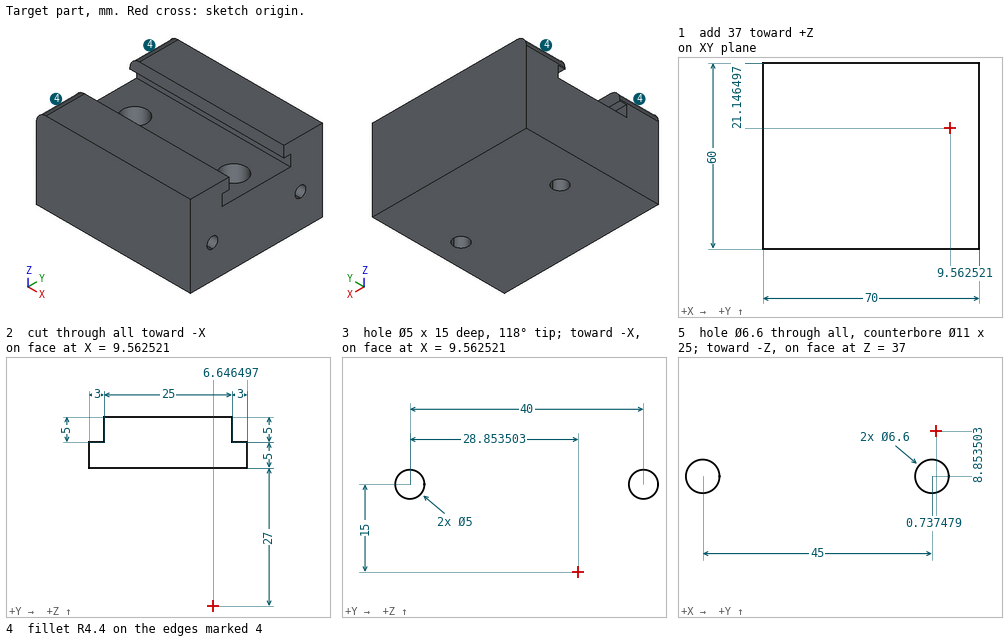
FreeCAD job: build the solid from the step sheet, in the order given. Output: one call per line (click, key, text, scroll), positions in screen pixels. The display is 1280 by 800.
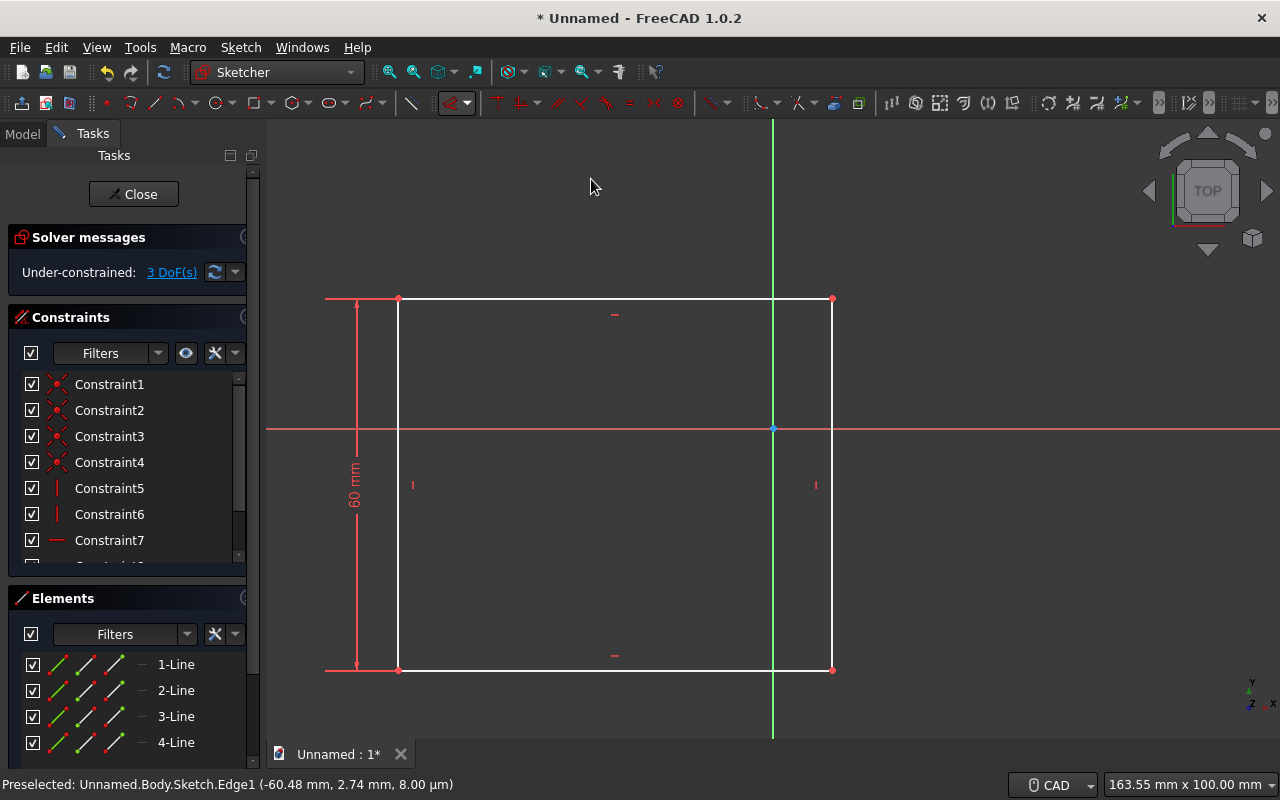
click(528, 671)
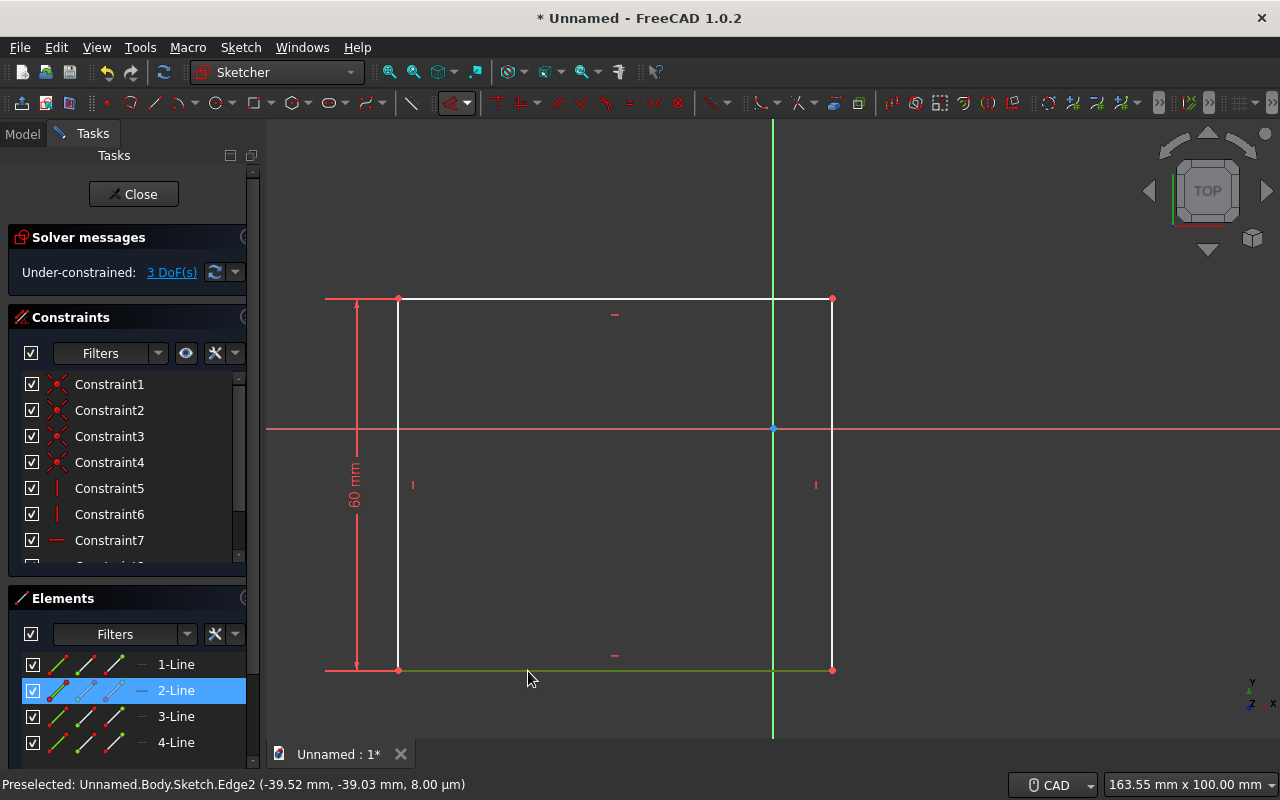
click(470, 104)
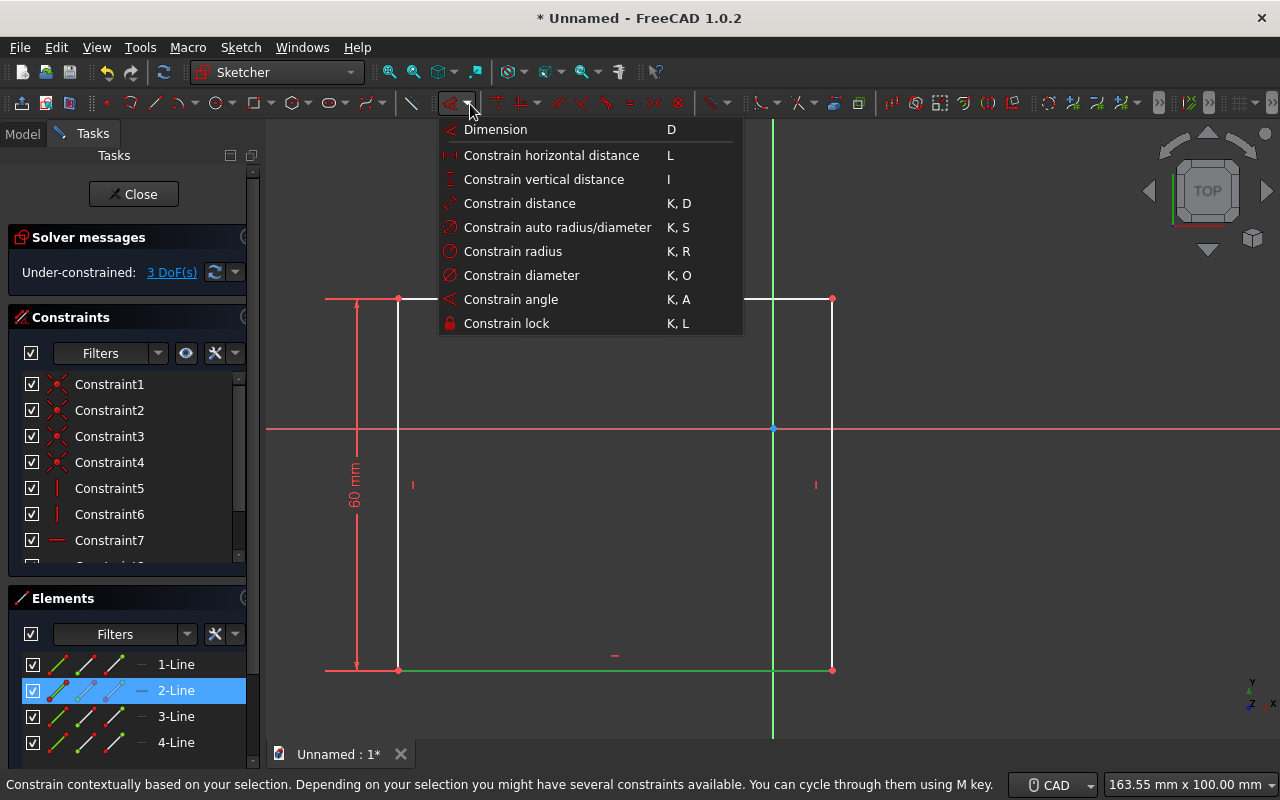
click(591, 155)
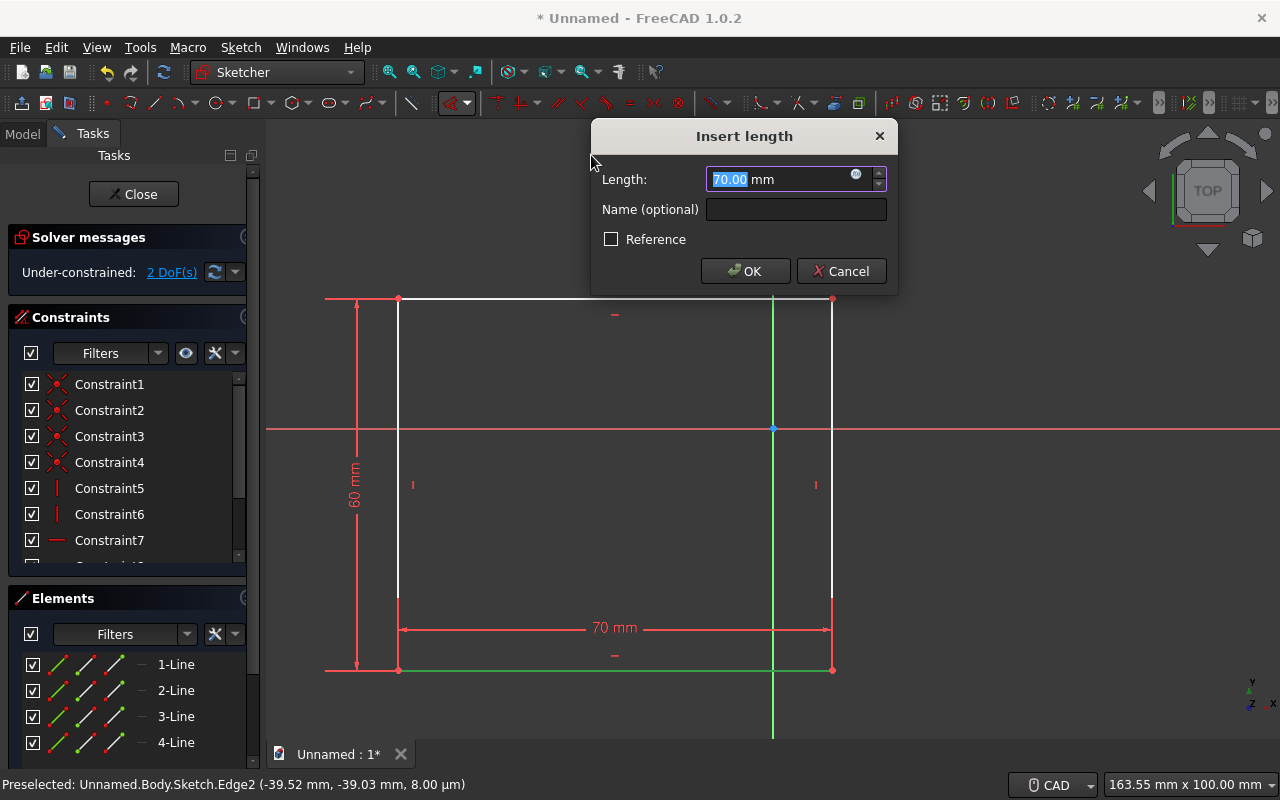
text(70)
key(Return)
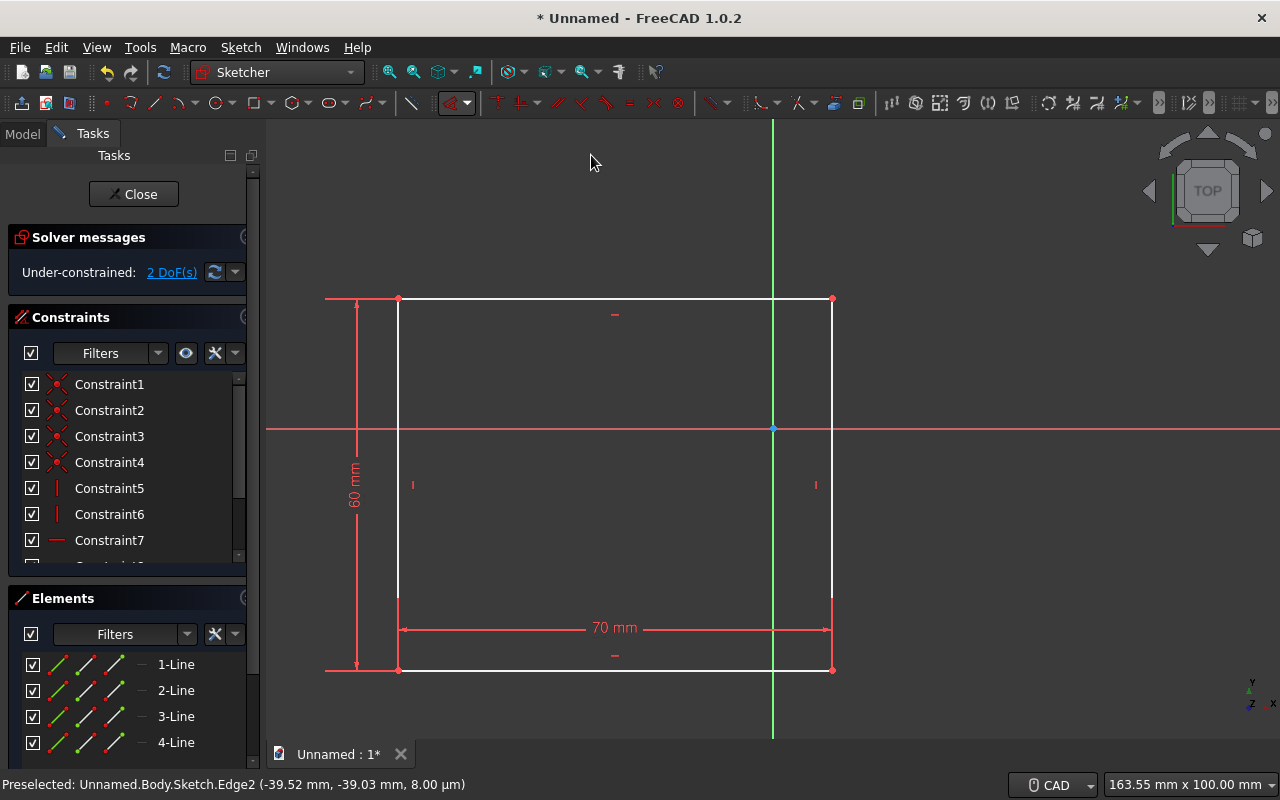
click(832, 671)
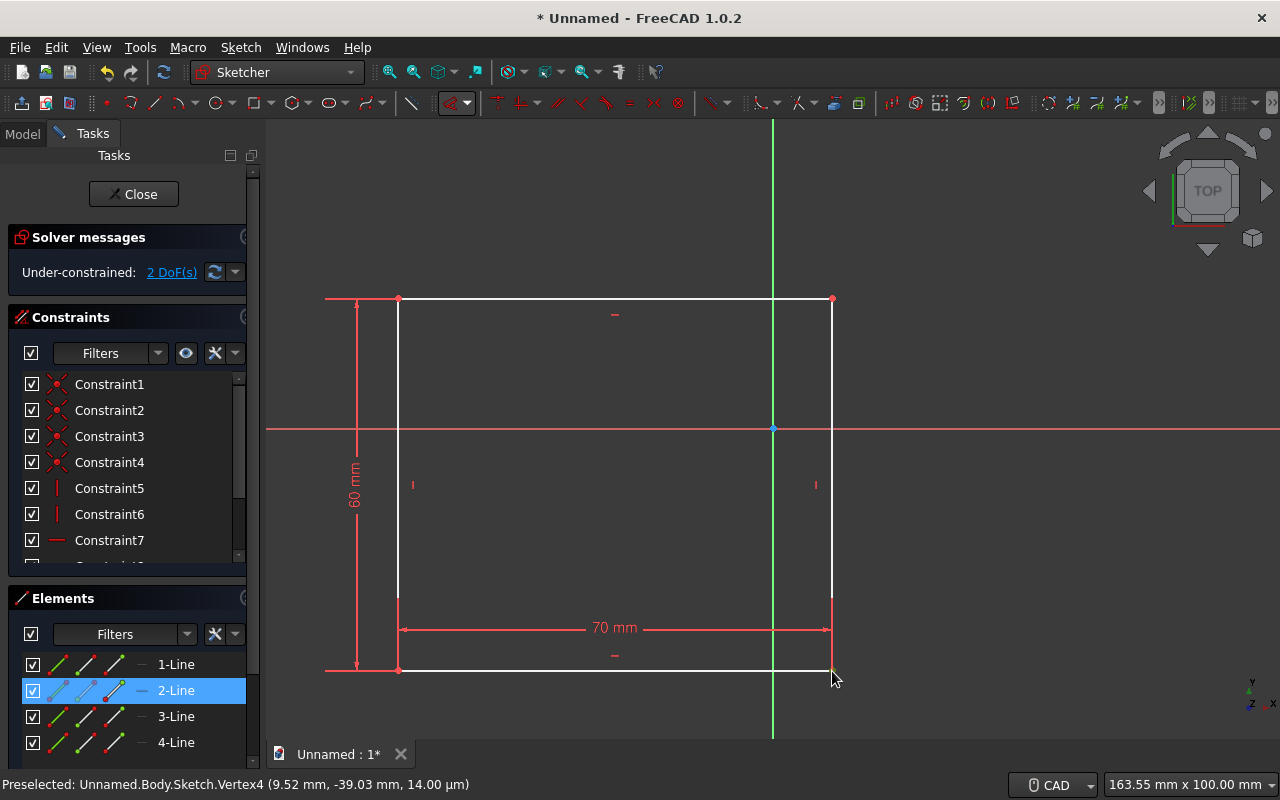
click(470, 104)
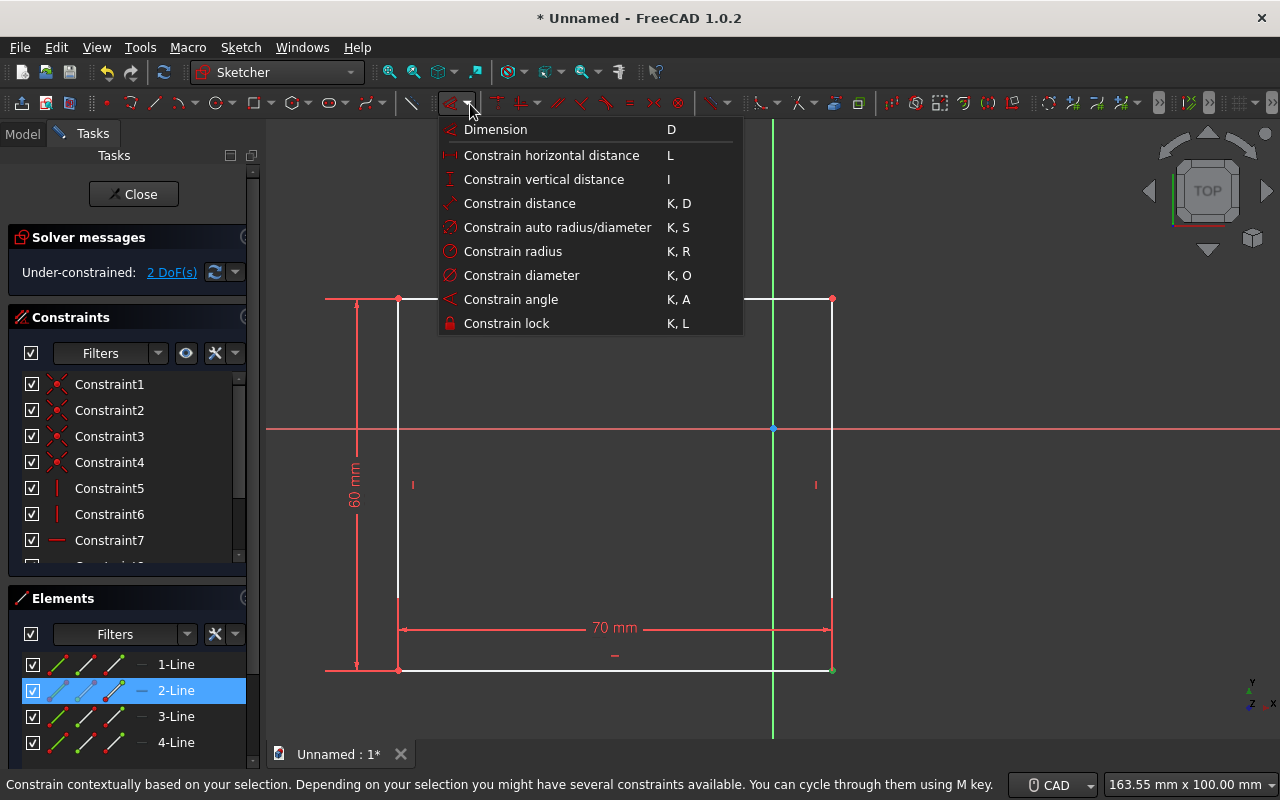
click(591, 155)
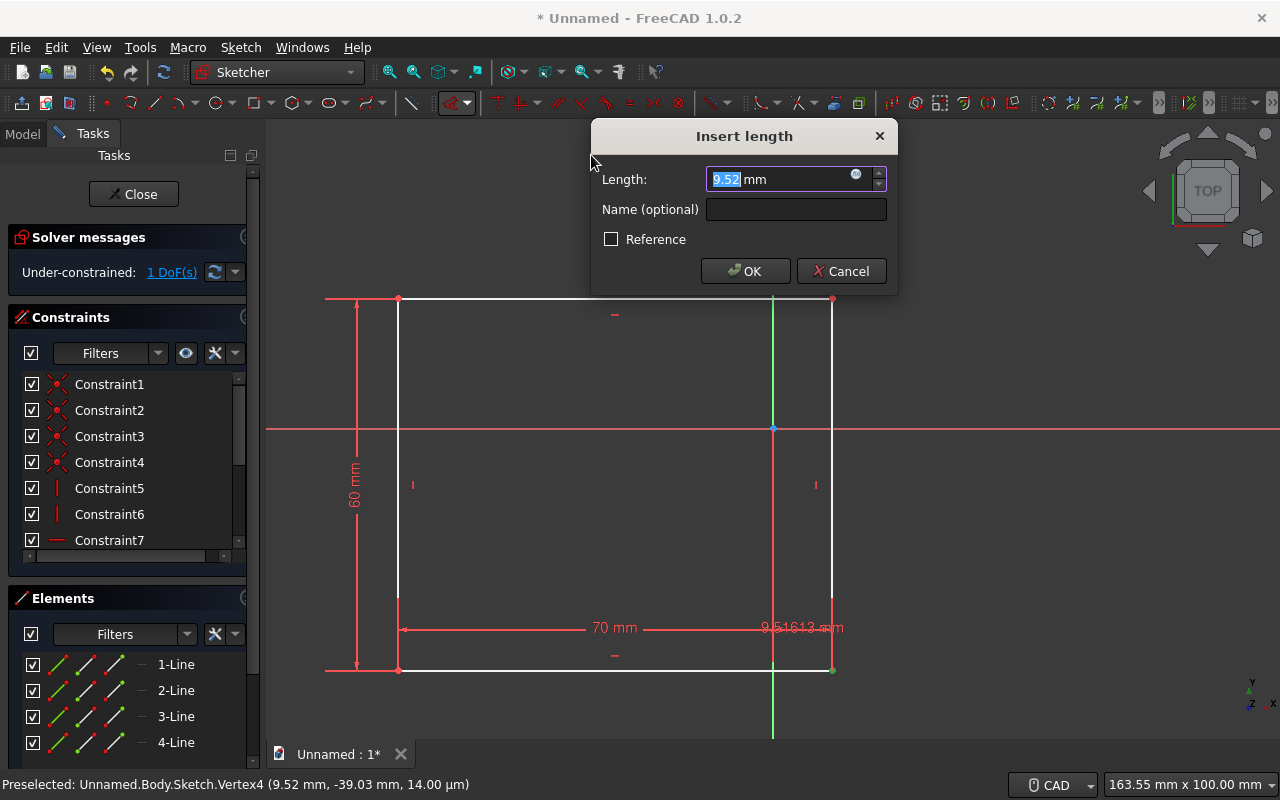
text(9.562521)
key(Return)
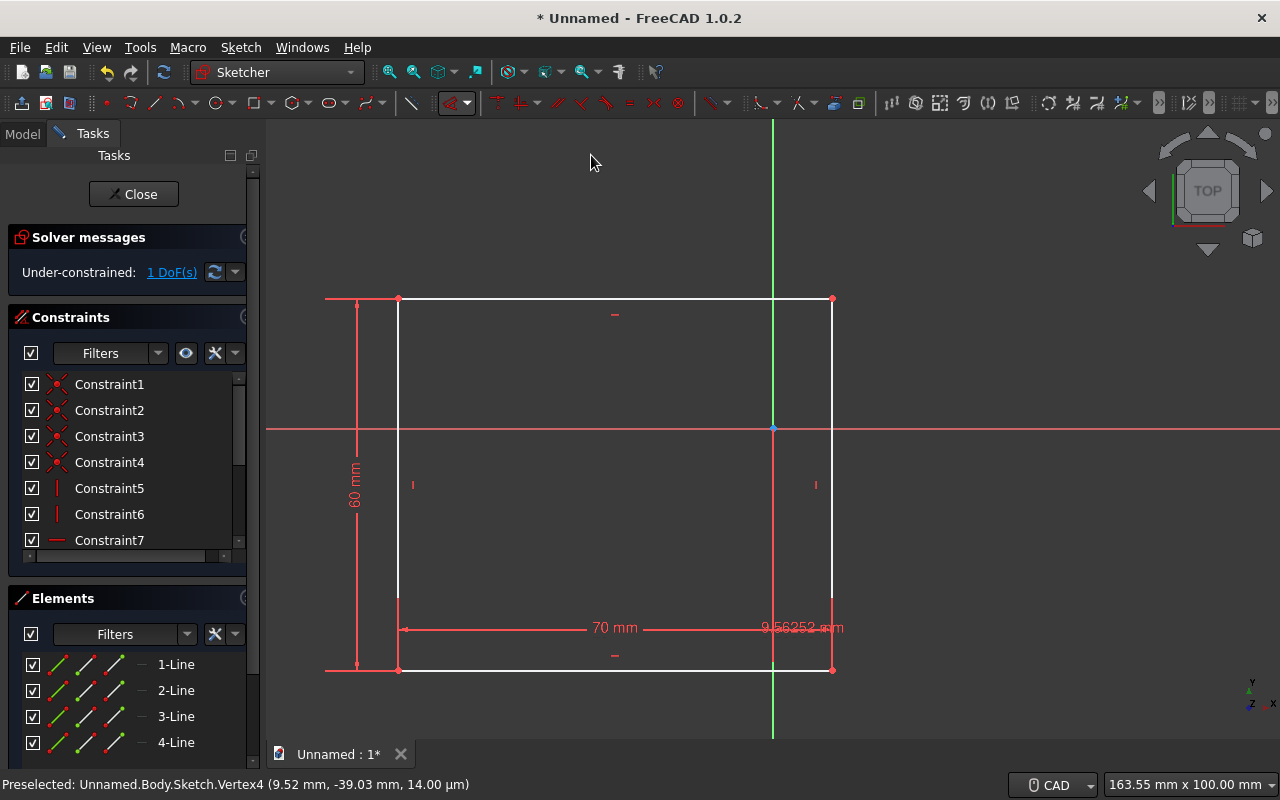
click(398, 299)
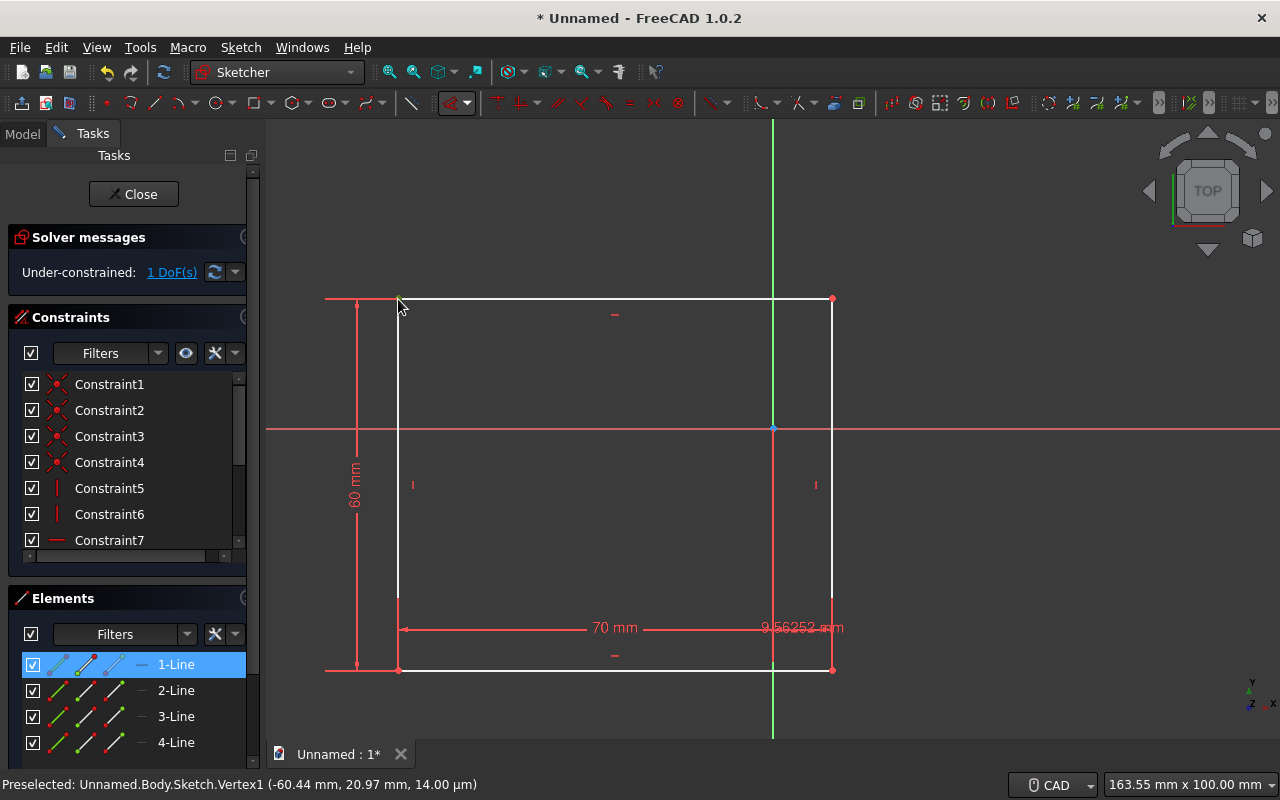
key(i)